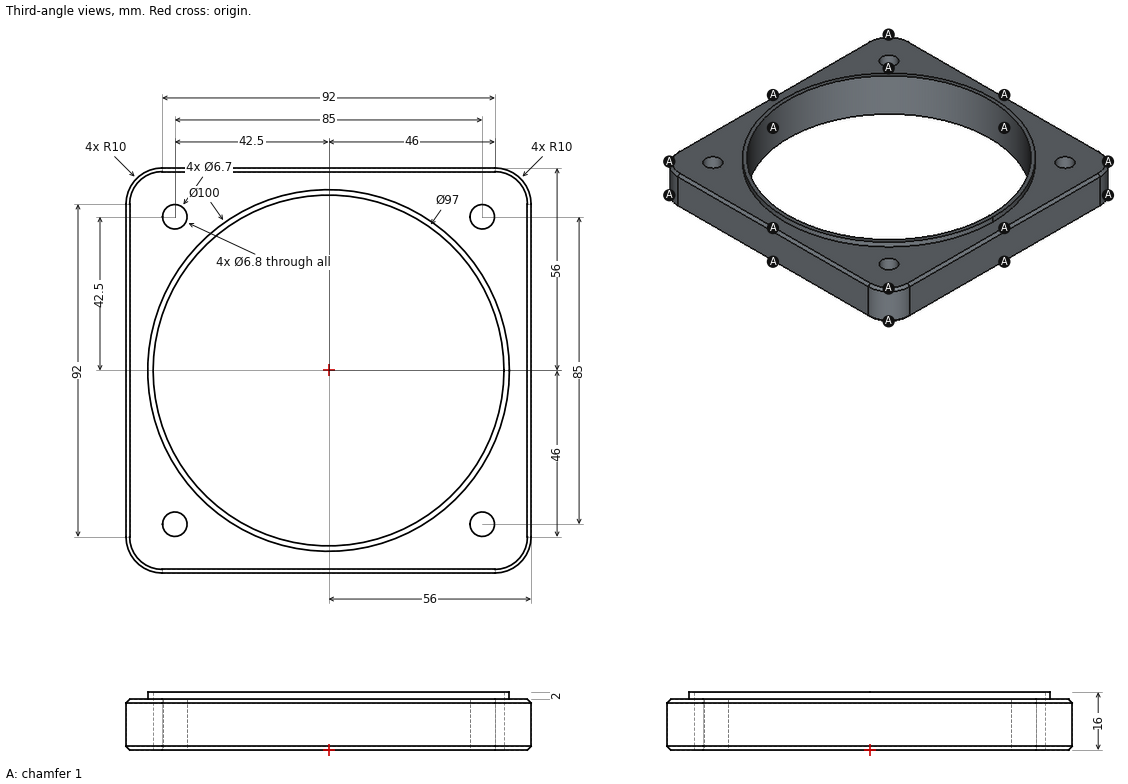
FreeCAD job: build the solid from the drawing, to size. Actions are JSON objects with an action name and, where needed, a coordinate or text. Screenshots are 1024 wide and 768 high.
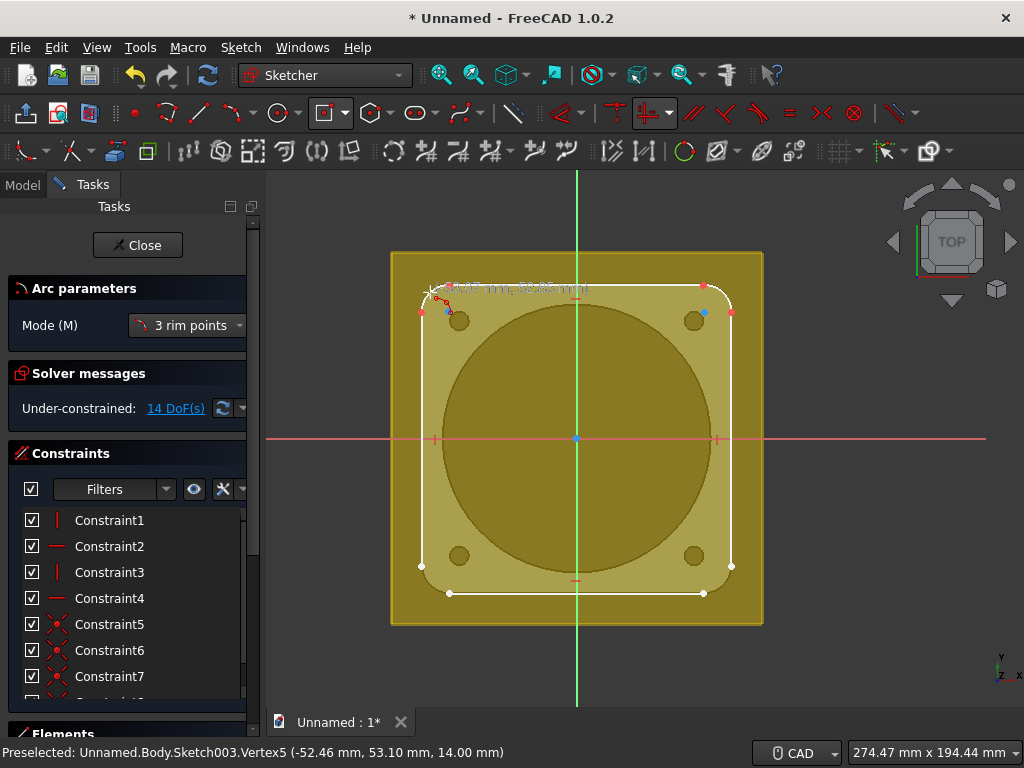
{"action": "left_click", "coordinate": [422, 567]}
{"action": "left_click", "coordinate": [450, 594]}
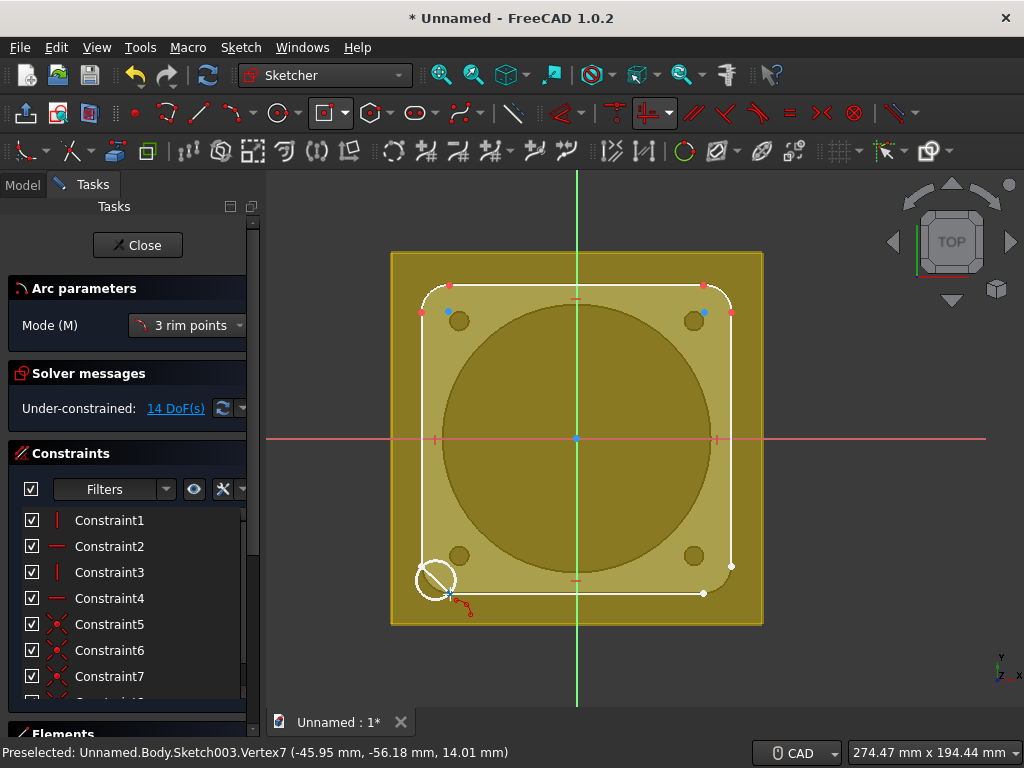
{"action": "scroll", "coordinate": [430, 585], "scroll_direction": "up", "scroll_amount": 4}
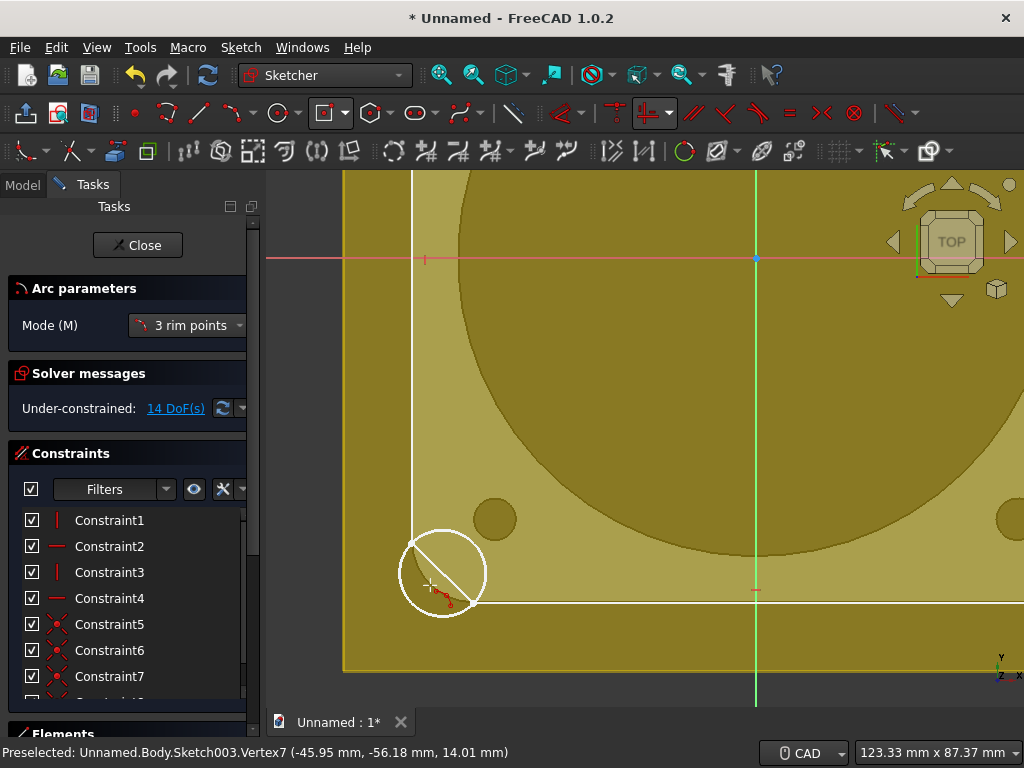
{"action": "left_click", "coordinate": [430, 584]}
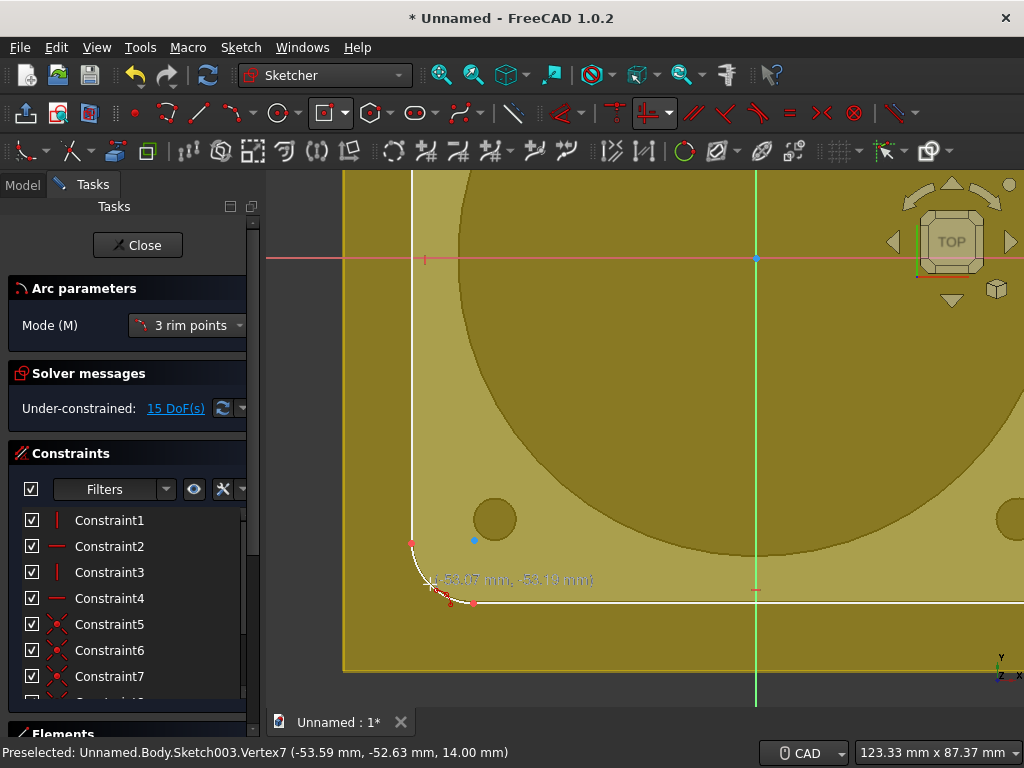
{"action": "scroll", "coordinate": [430, 586], "scroll_direction": "down", "scroll_amount": 4}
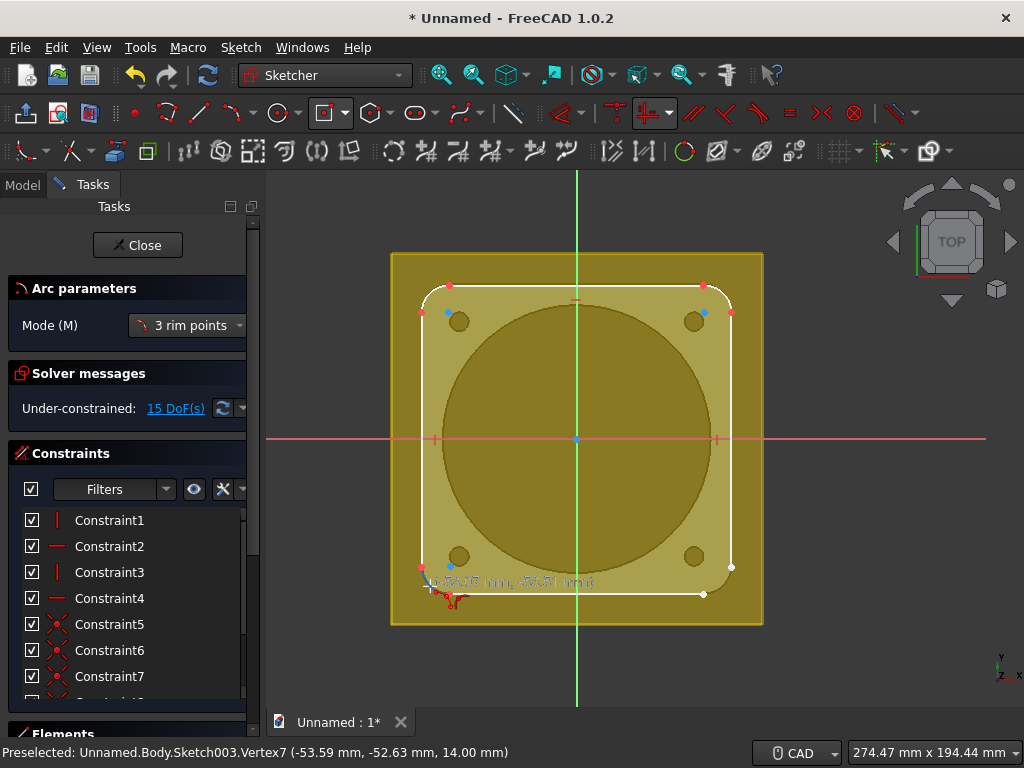
{"action": "left_click", "coordinate": [704, 594]}
{"action": "left_click", "coordinate": [731, 567]}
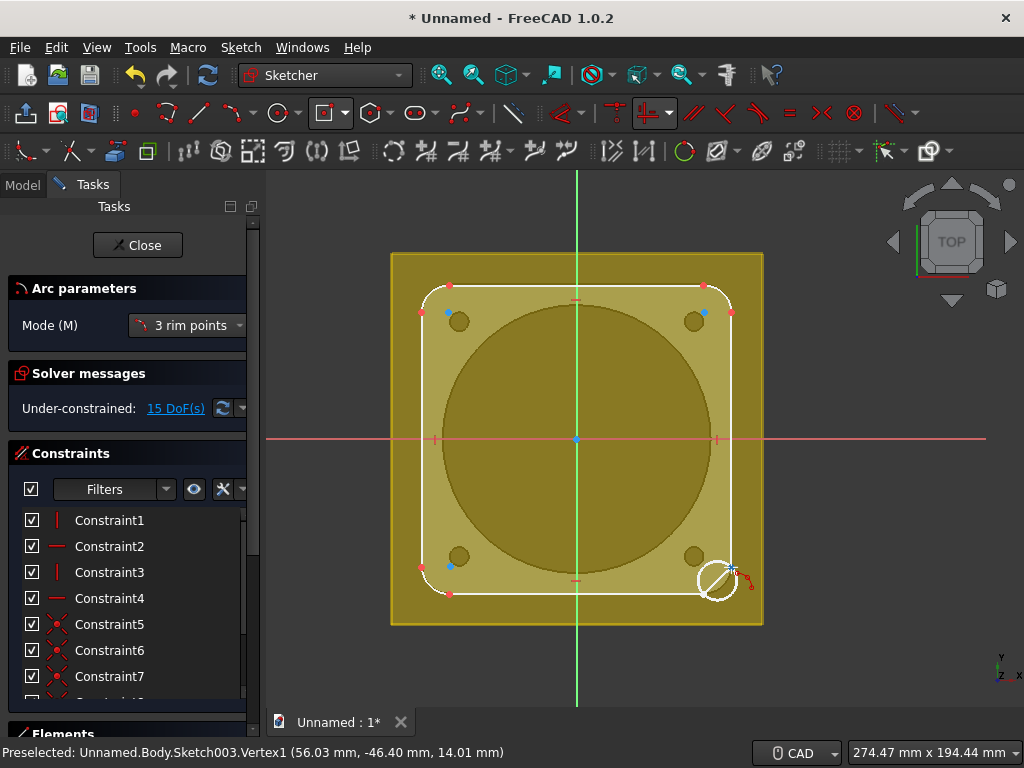
{"action": "scroll", "coordinate": [723, 586], "scroll_direction": "up", "scroll_amount": 4}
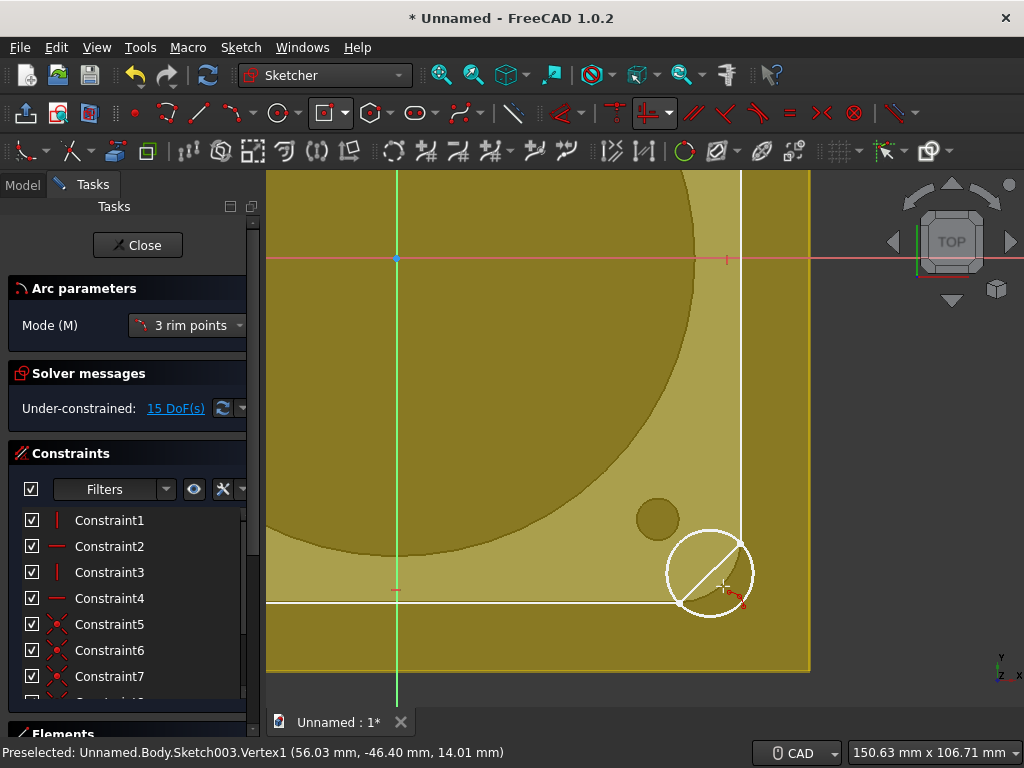
{"action": "left_click", "coordinate": [723, 584]}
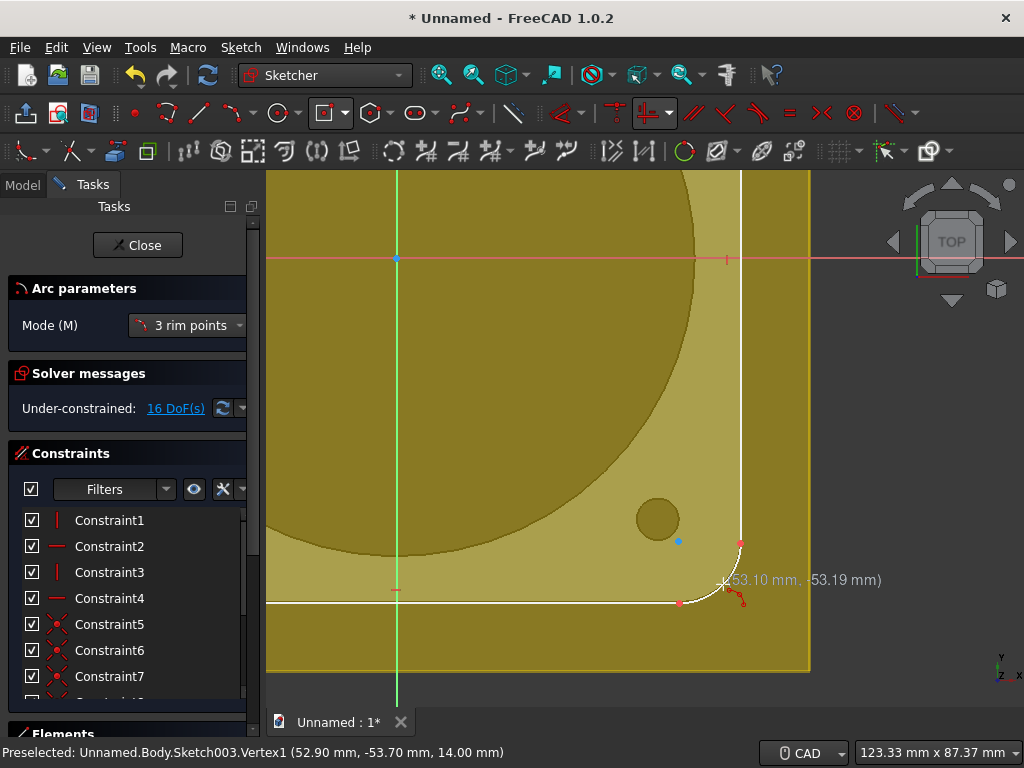
{"action": "left_click", "coordinate": [278, 114]}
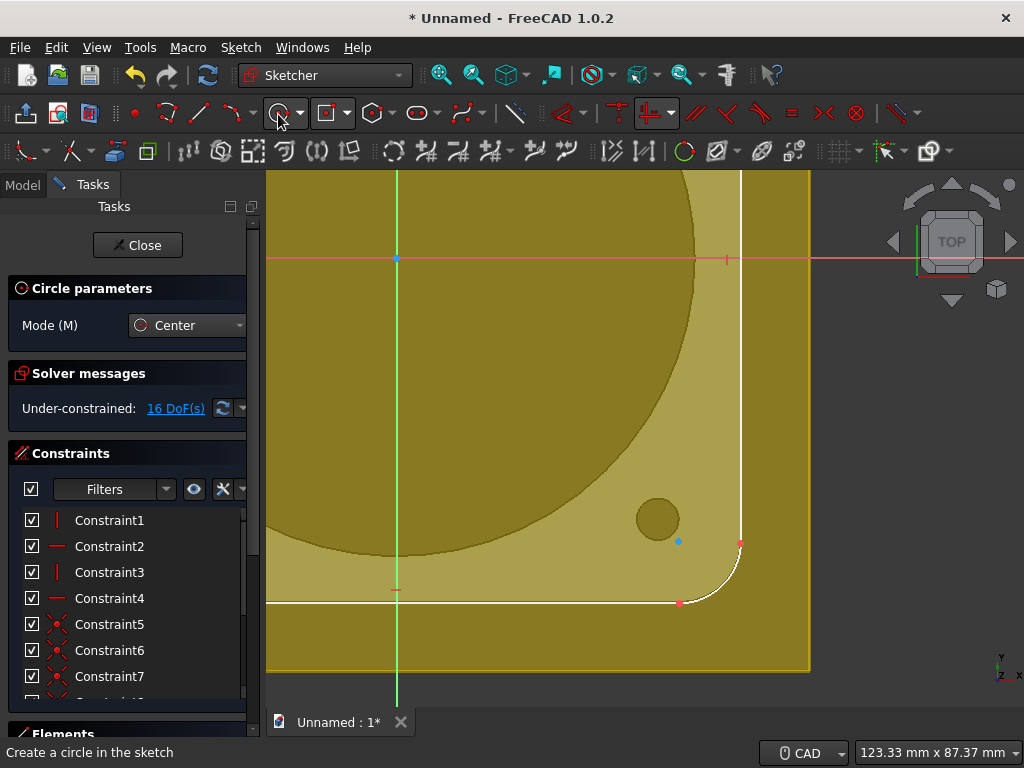
{"action": "left_click", "coordinate": [397, 258]}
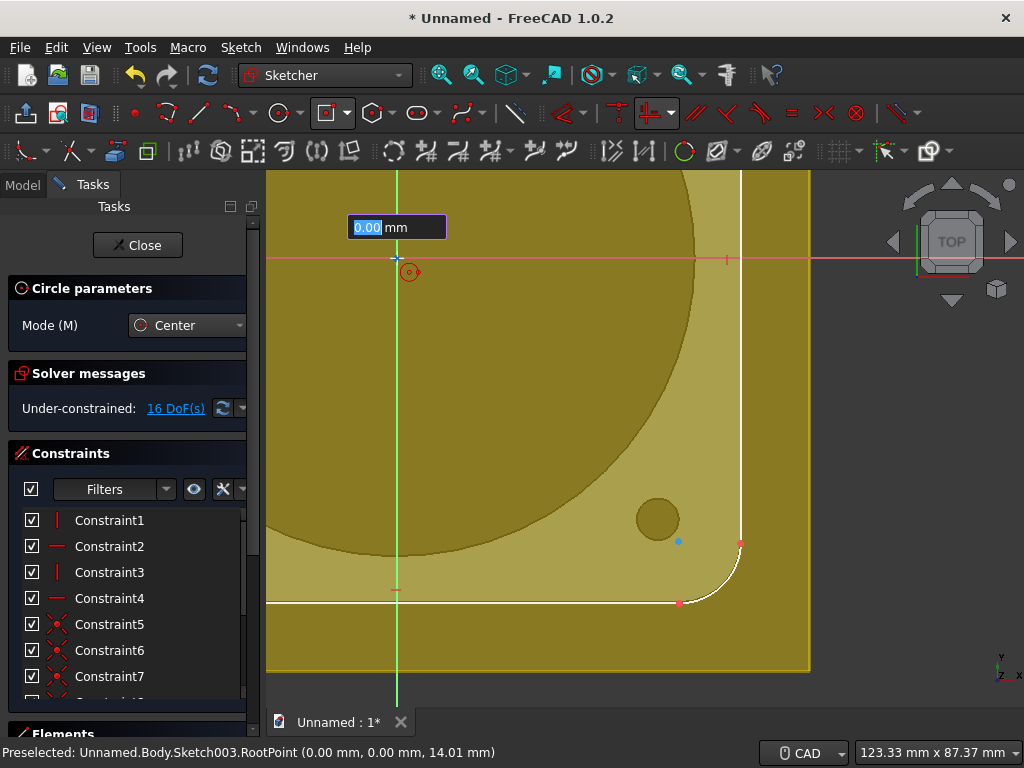
{"action": "scroll", "coordinate": [723, 586], "scroll_direction": "down", "scroll_amount": 4}
{"action": "mouse_move", "coordinate": [674, 341]}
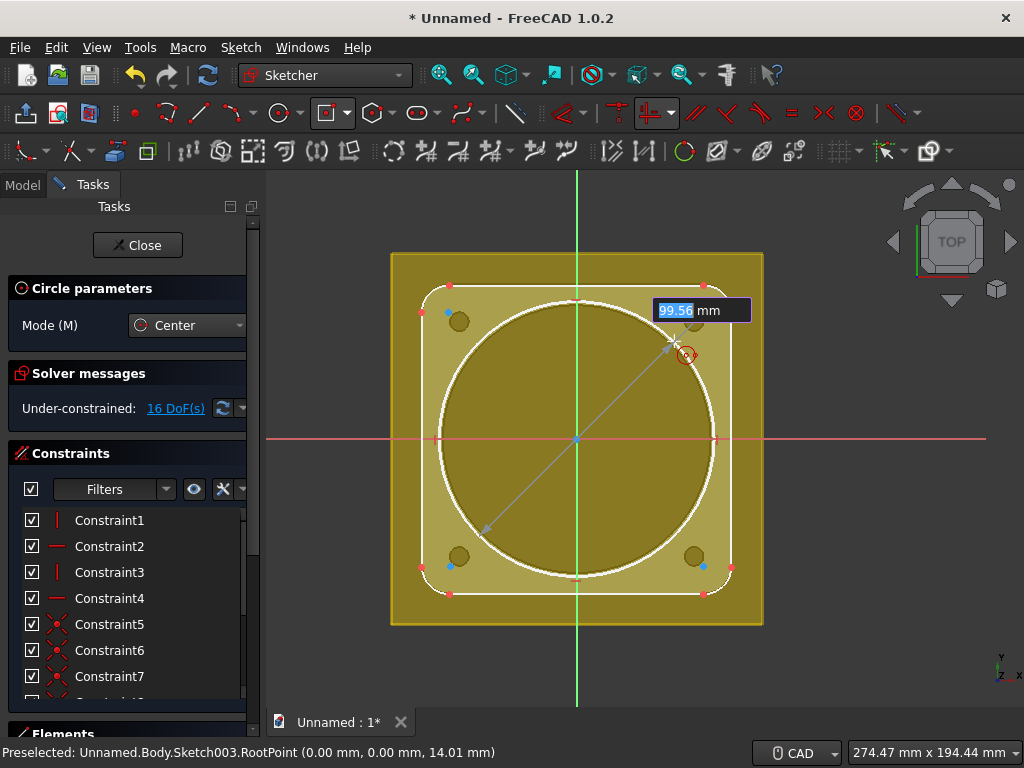
{"action": "type", "text": "100"}
{"action": "key", "text": "Return"}
{"action": "key", "text": "Escape"}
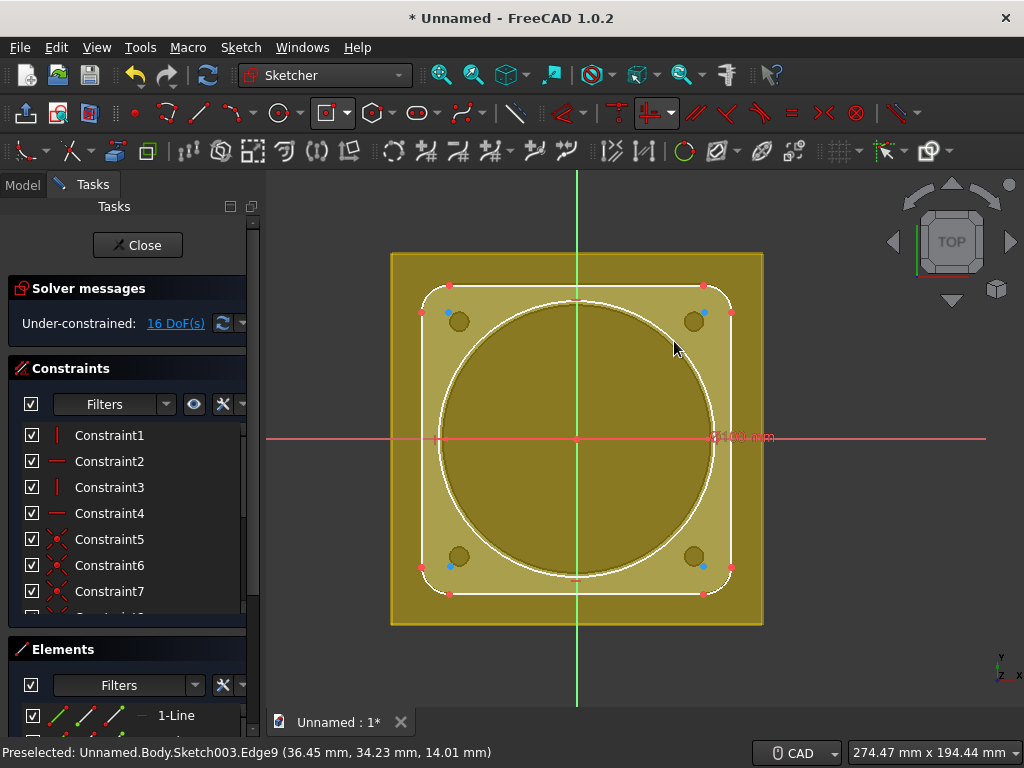
{"action": "left_click", "coordinate": [731, 491]}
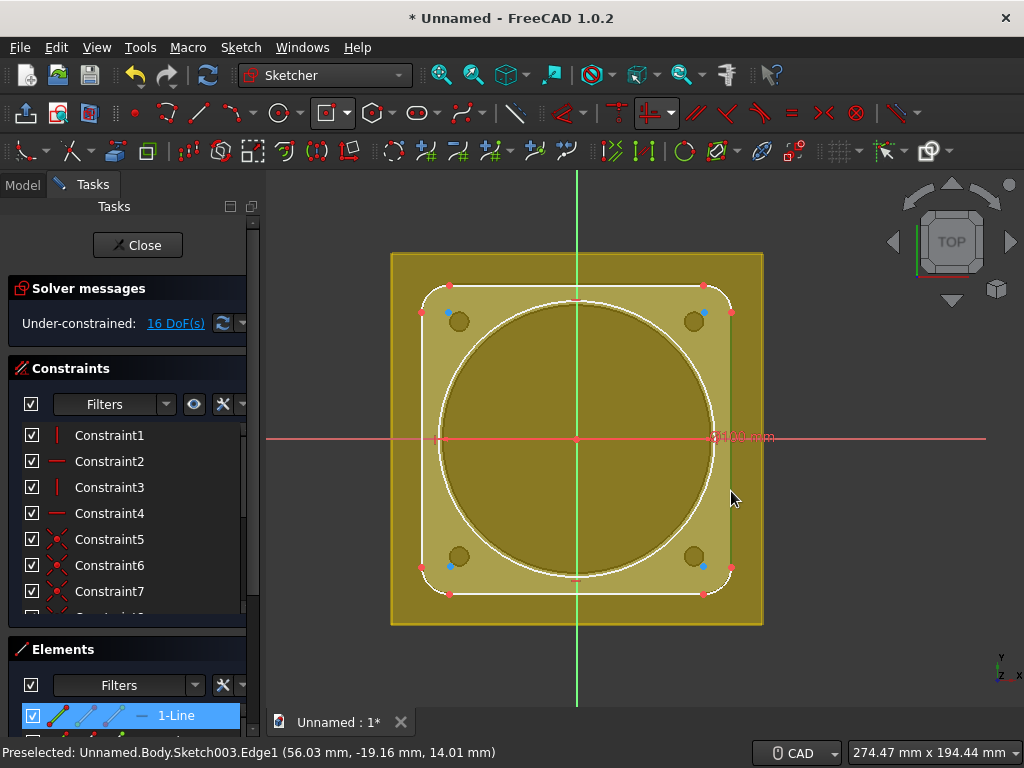
{"action": "left_click", "coordinate": [728, 300]}